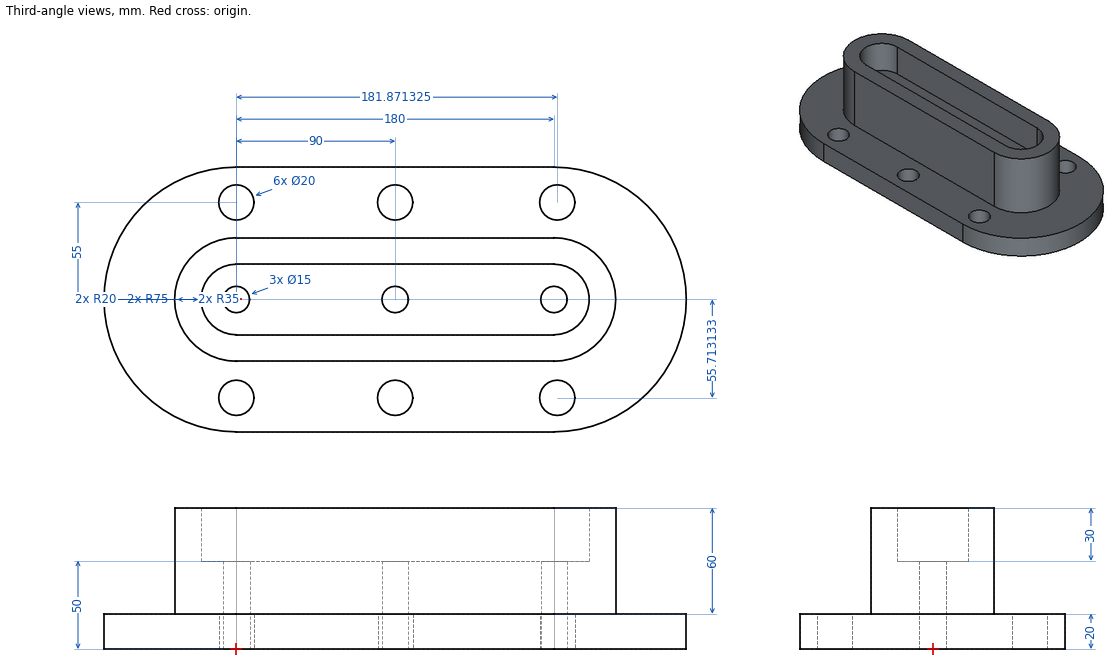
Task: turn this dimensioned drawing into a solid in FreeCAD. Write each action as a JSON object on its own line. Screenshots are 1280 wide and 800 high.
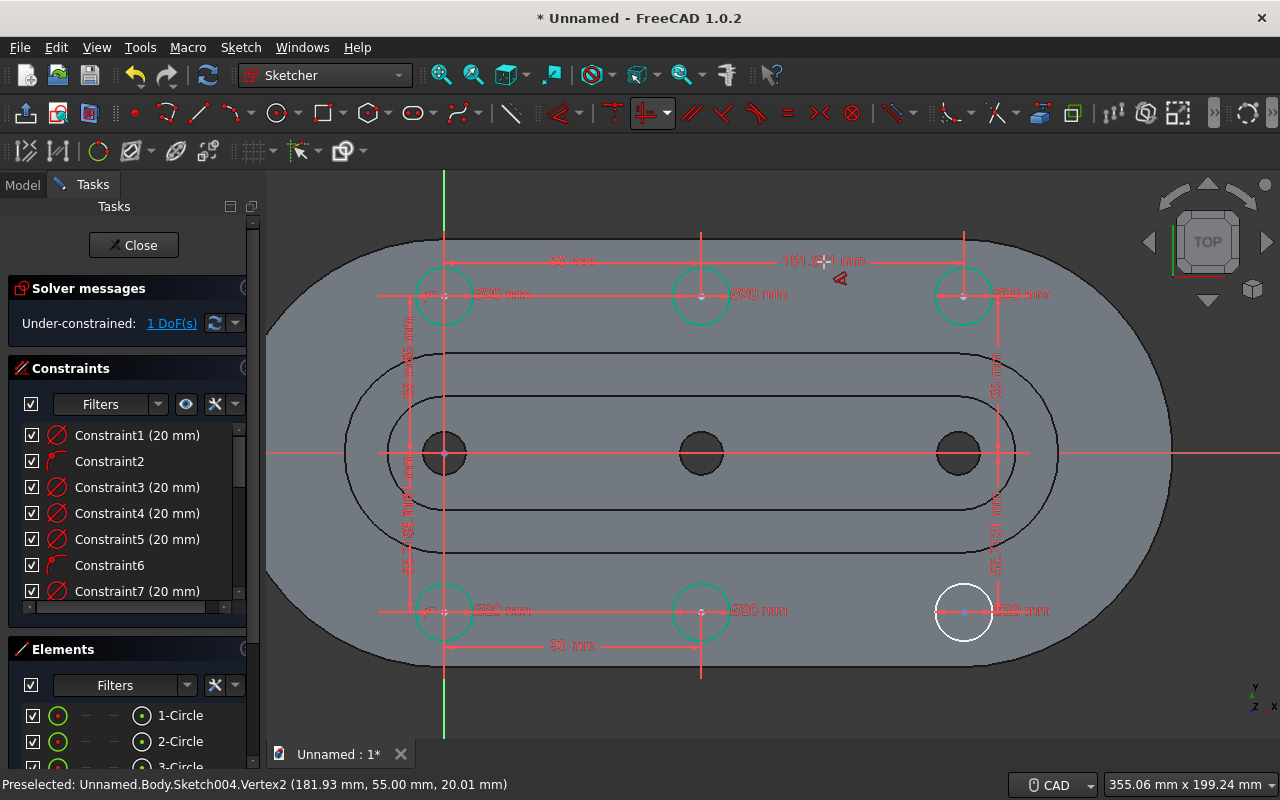
{"action": "left_click", "coordinate": [964, 612]}
{"action": "left_click", "coordinate": [824, 646]}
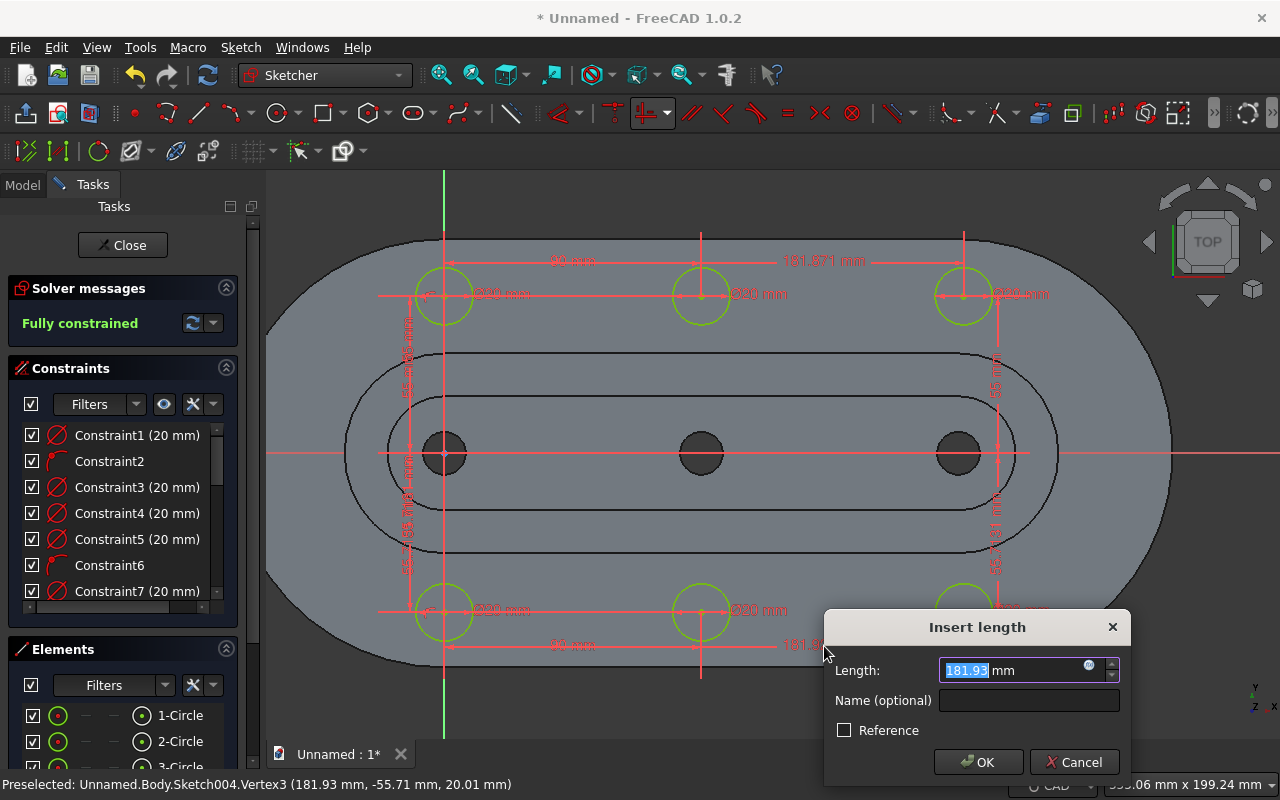
{"action": "type", "text": "181.871325"}
{"action": "key", "text": "Return"}
{"action": "key", "text": "Escape"}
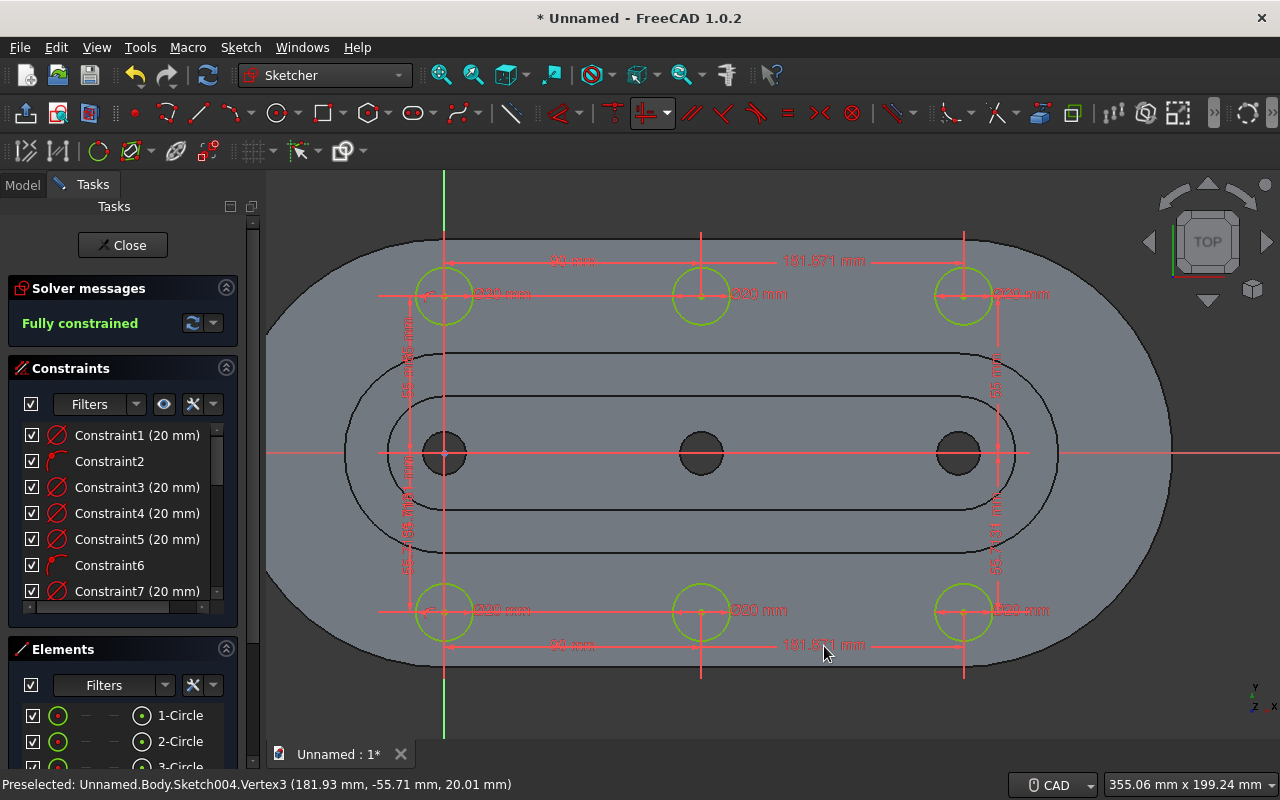
{"action": "left_click", "coordinate": [123, 245]}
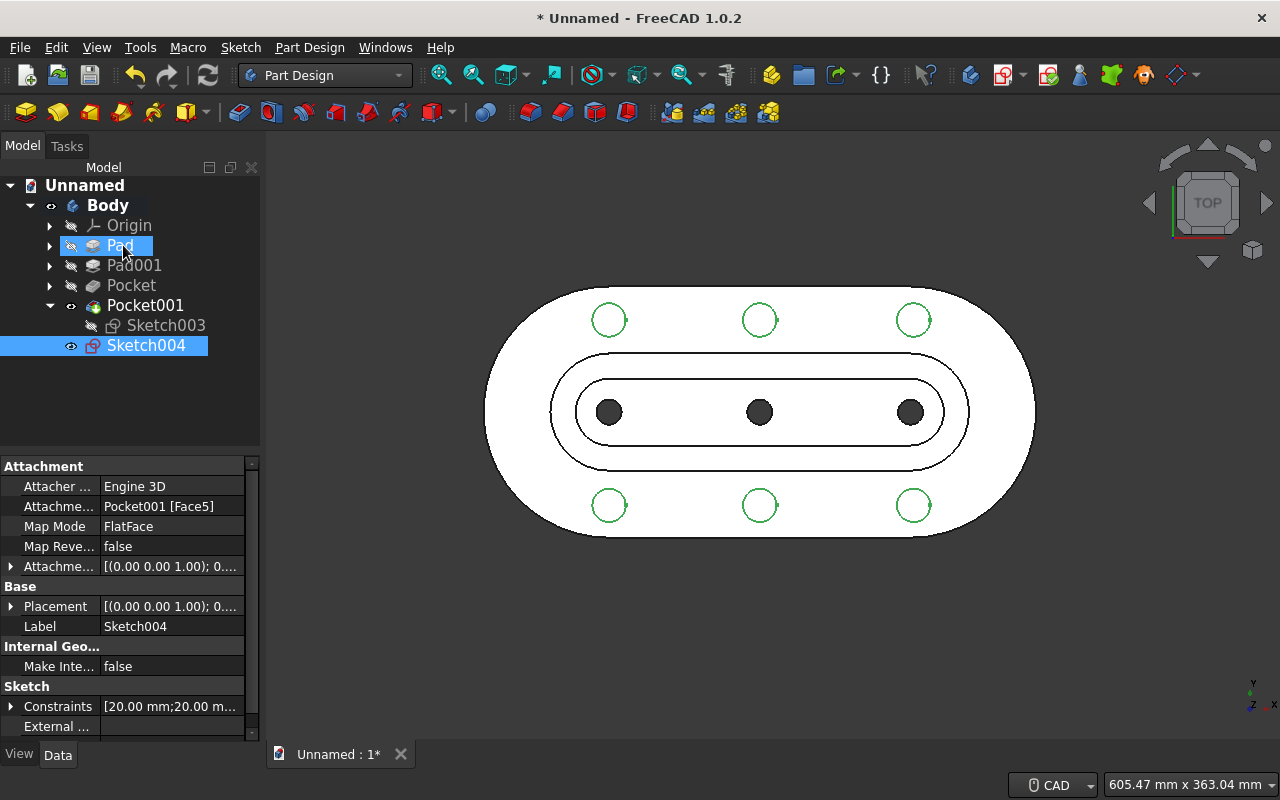
{"action": "left_click", "coordinate": [240, 112]}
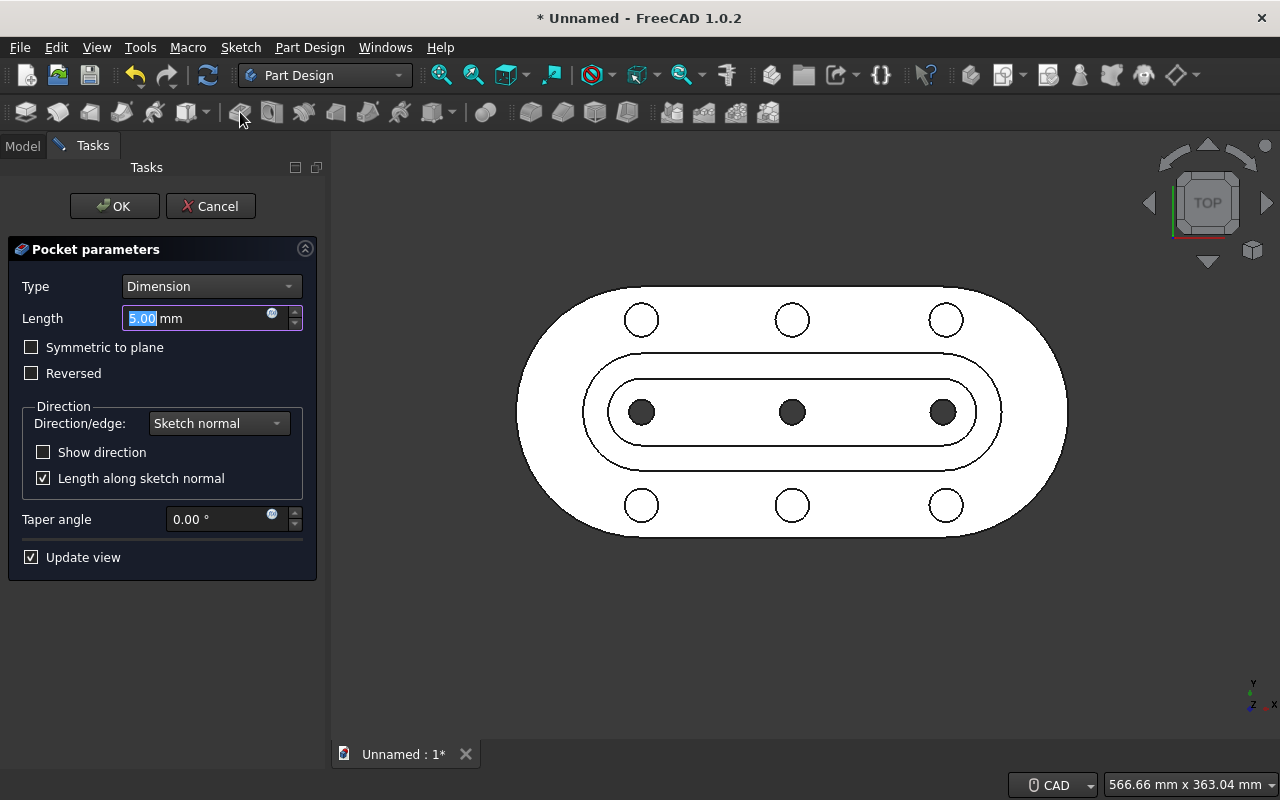
{"action": "type", "text": "20"}
{"action": "key", "text": "Tab"}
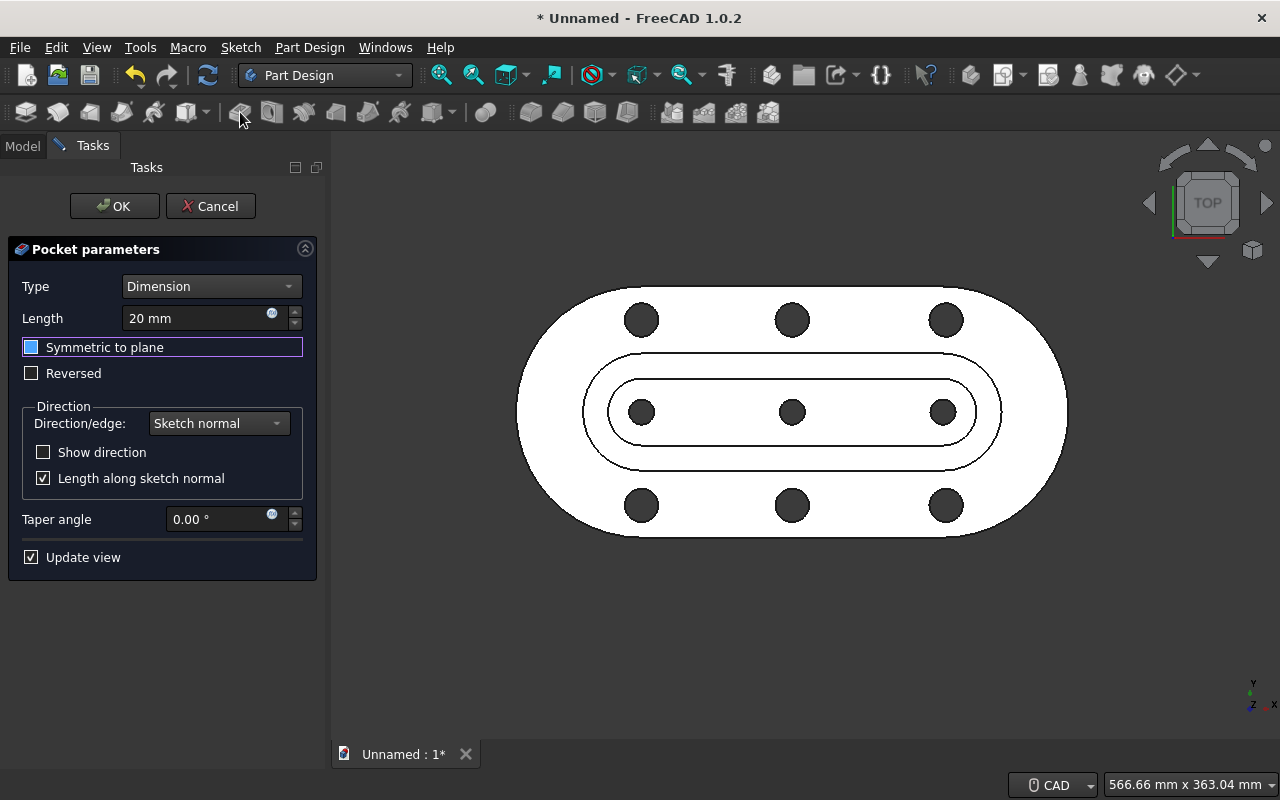
{"action": "left_click", "coordinate": [115, 206]}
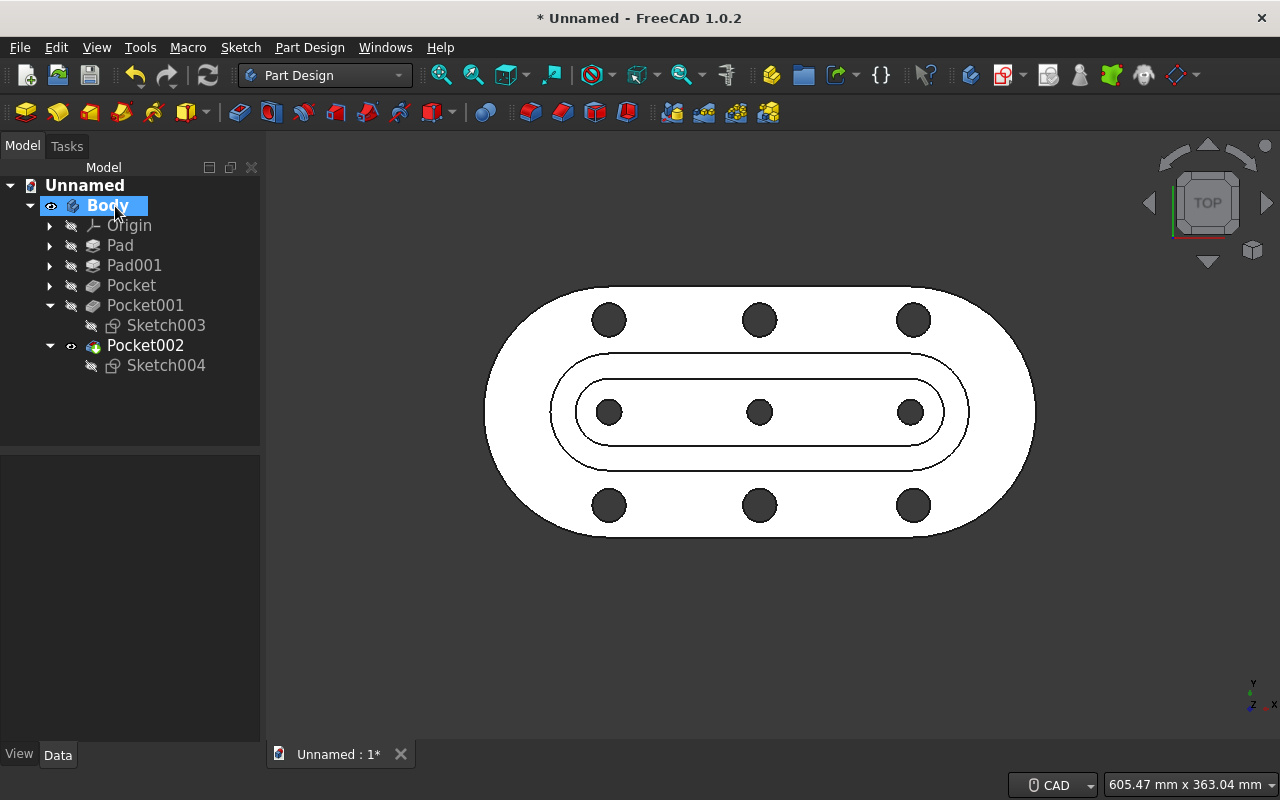
{"action": "key", "text": "0"}